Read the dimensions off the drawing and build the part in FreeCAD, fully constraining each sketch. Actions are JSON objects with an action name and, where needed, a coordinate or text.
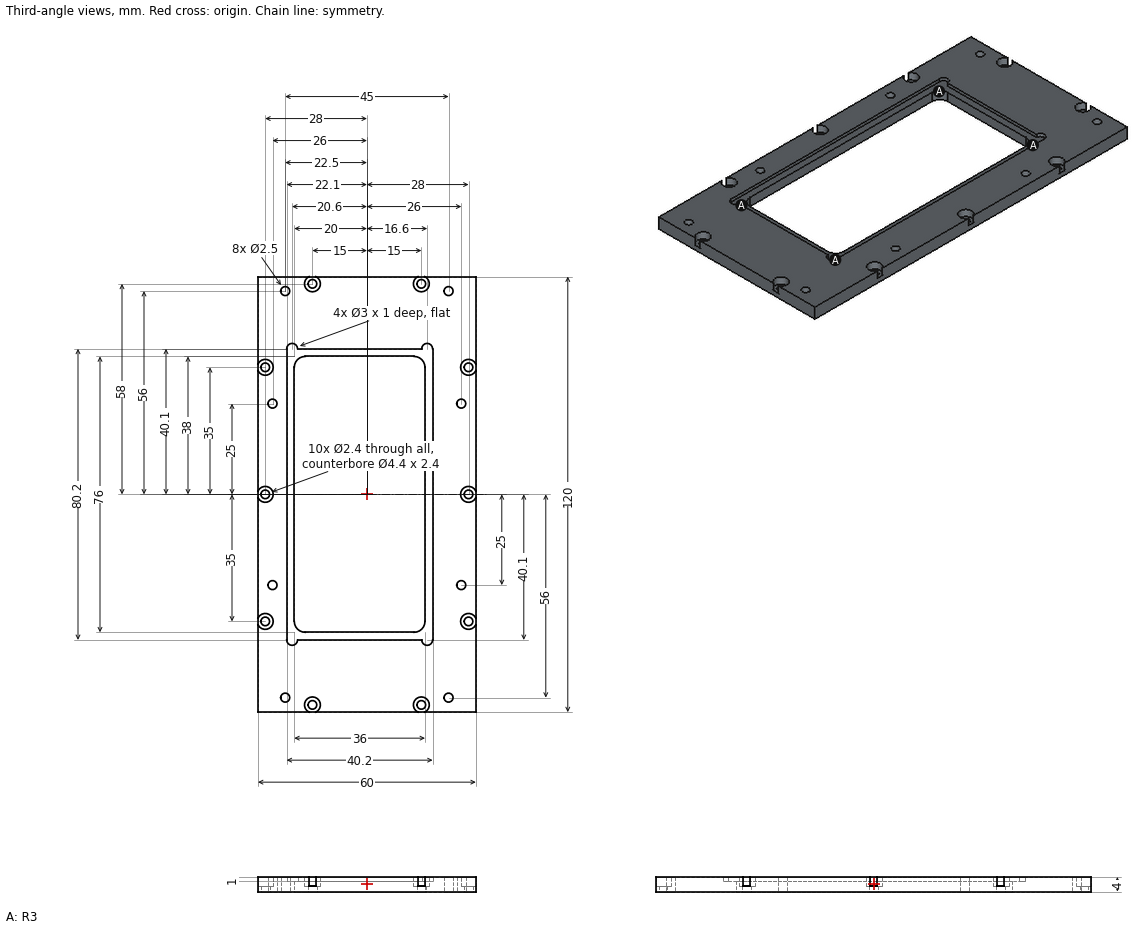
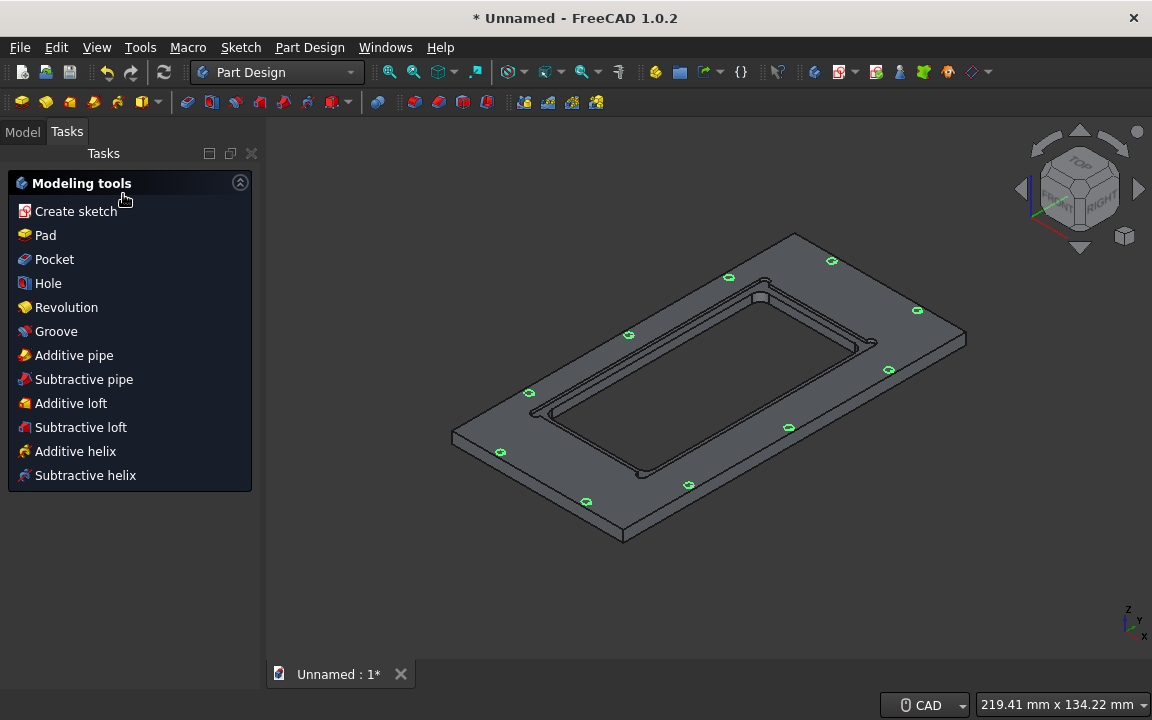
{"action": "left_click", "coordinate": [212, 102]}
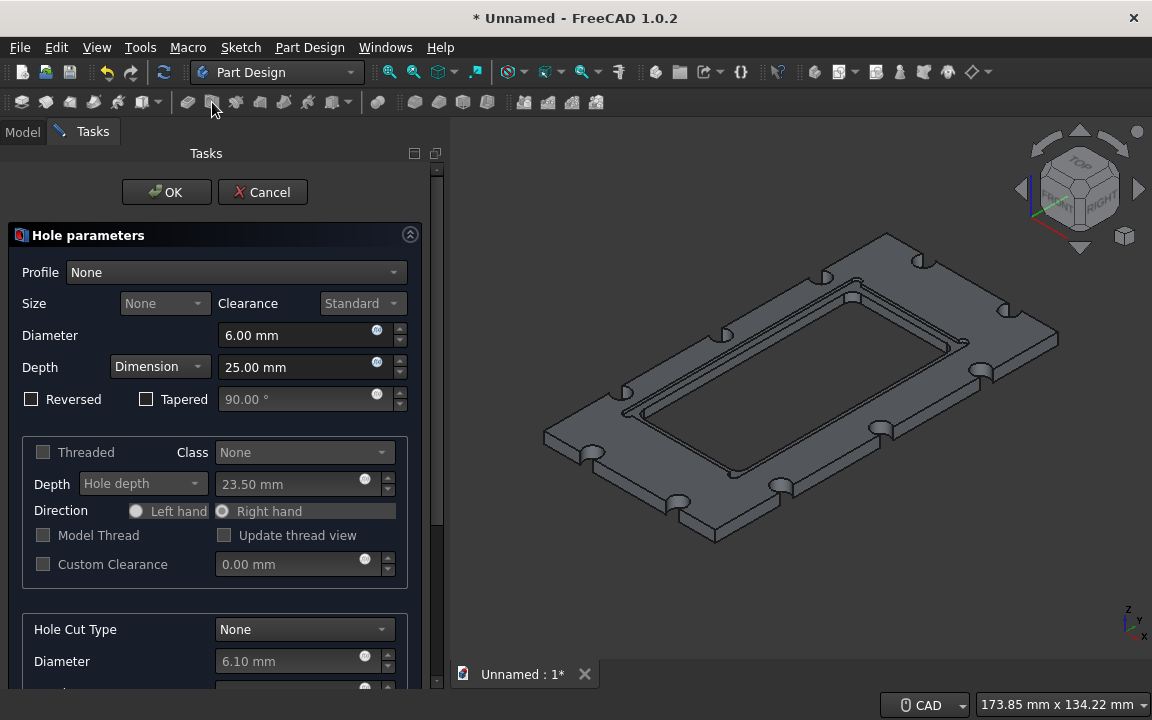
{"action": "triple_click", "coordinate": [305, 335]}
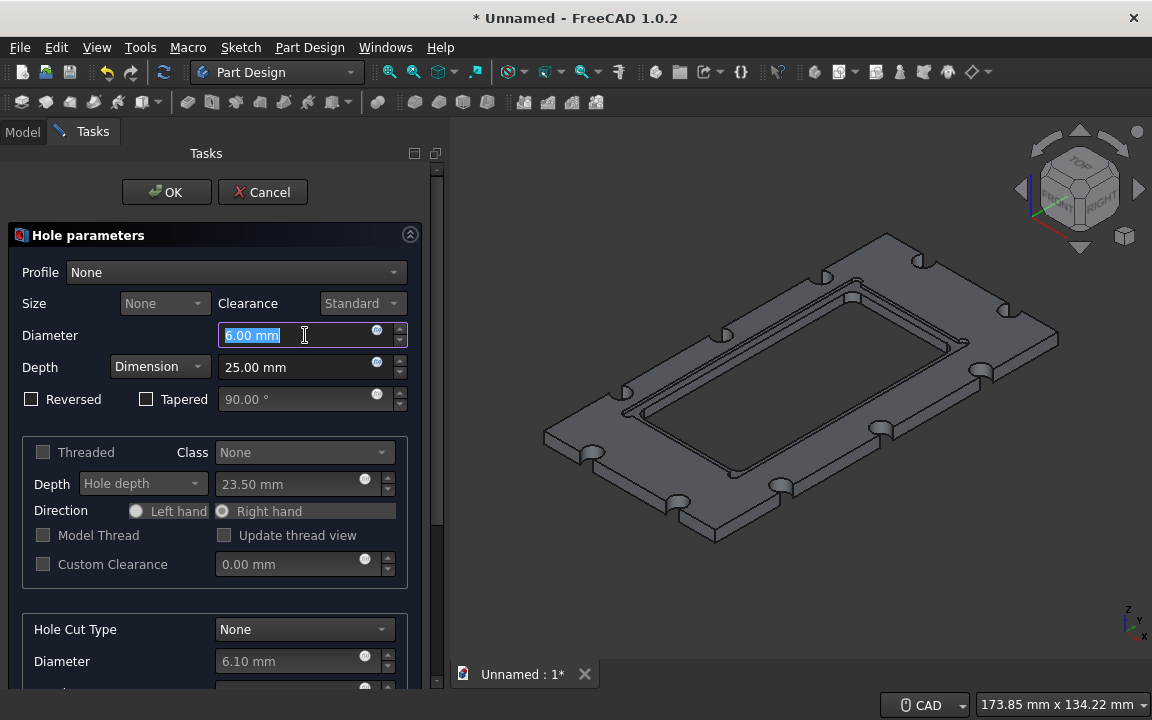
{"action": "type", "text": "2.4"}
{"action": "key", "text": "Tab"}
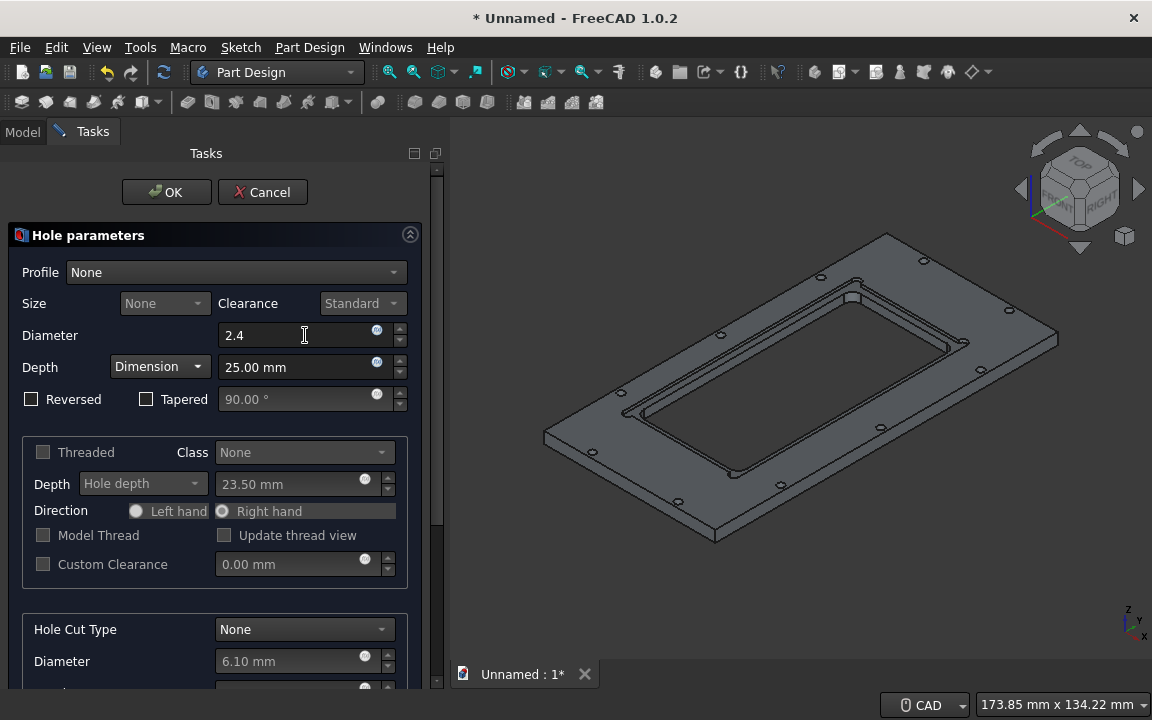
{"action": "left_click", "coordinate": [161, 366]}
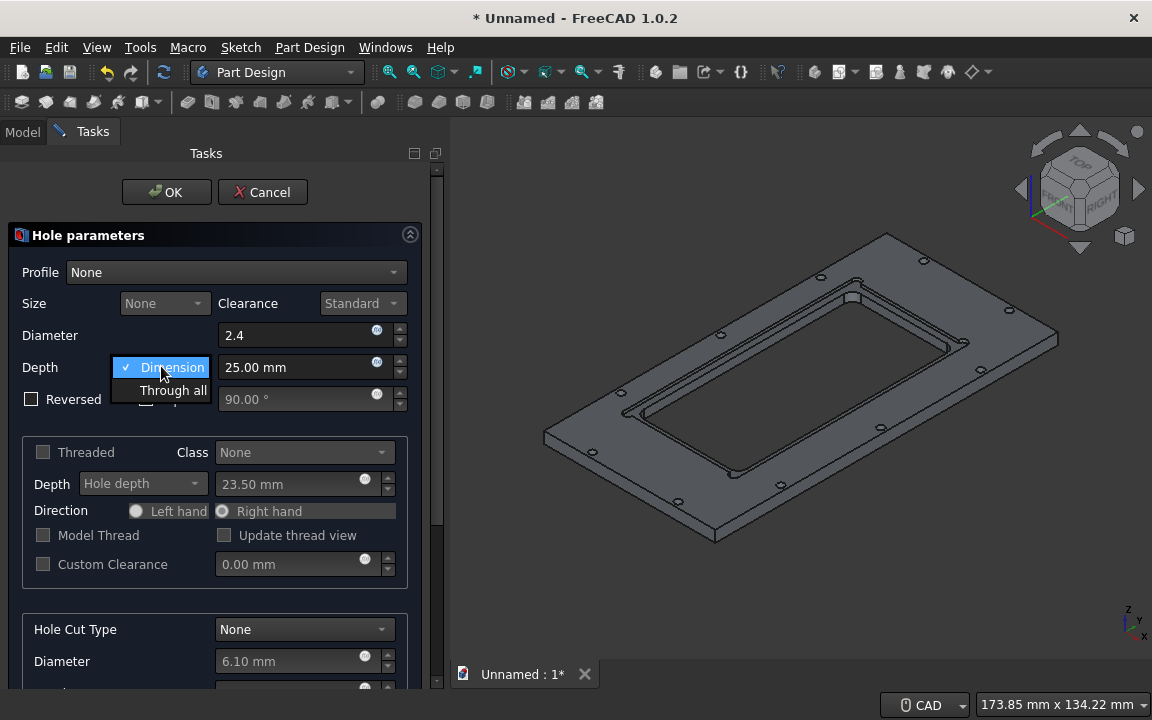
{"action": "left_click", "coordinate": [160, 390]}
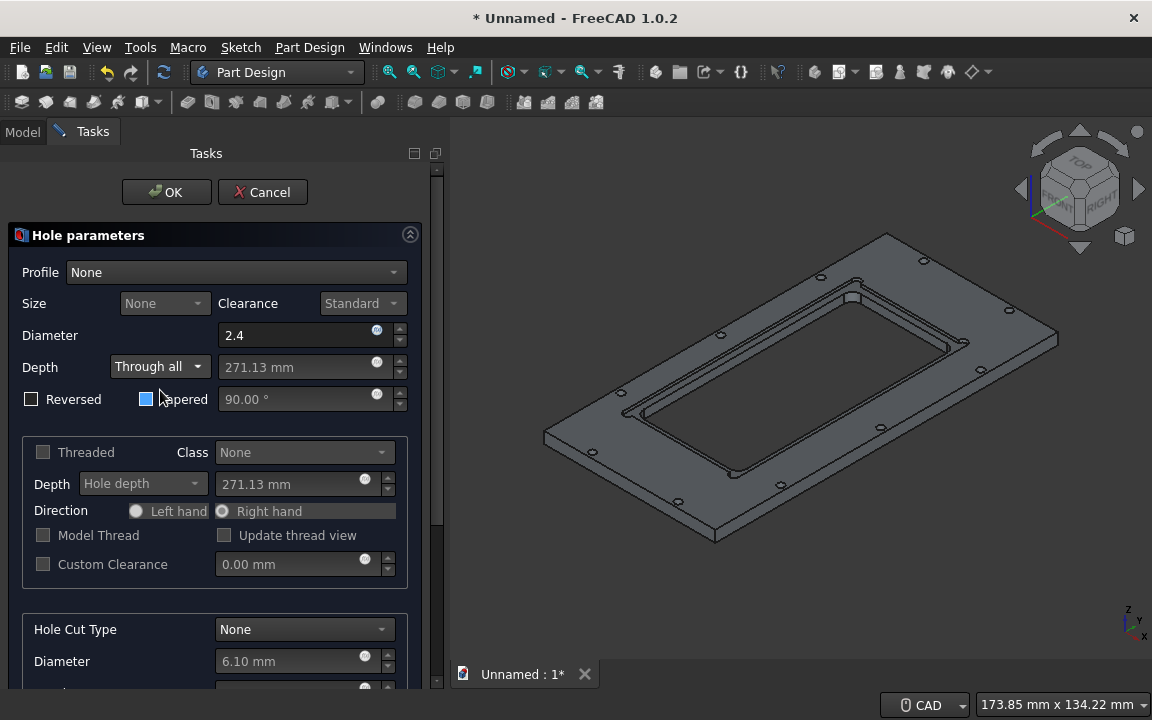
{"action": "left_click", "coordinate": [306, 630]}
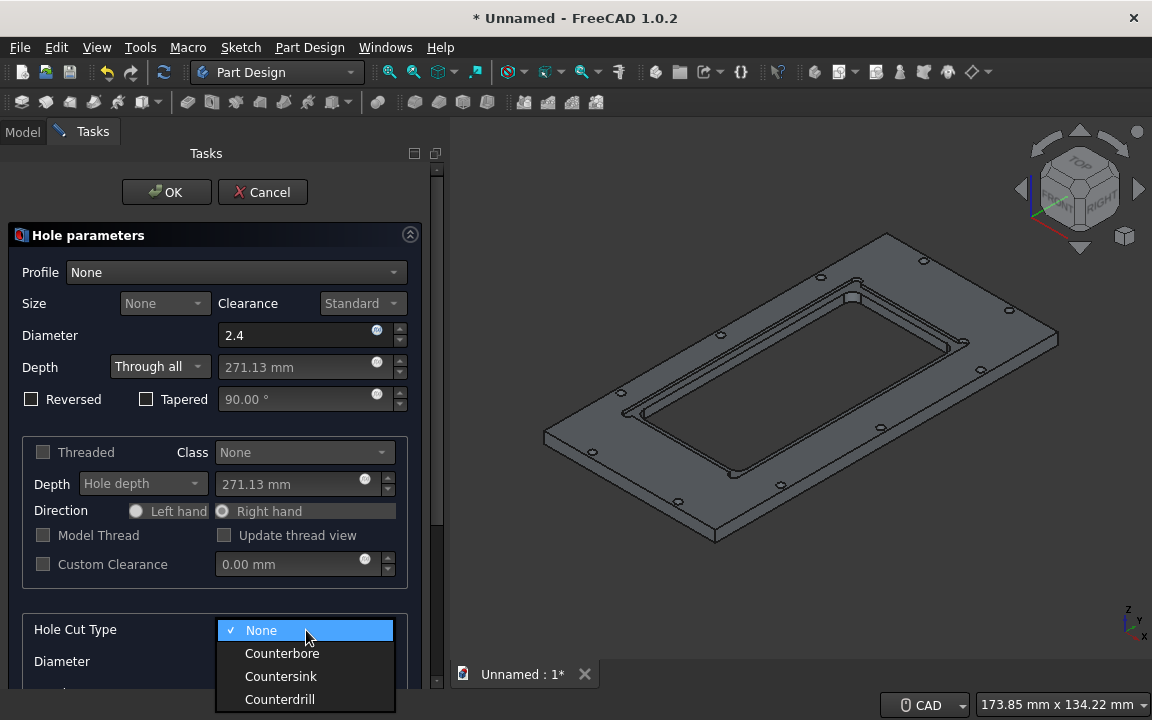
{"action": "left_click", "coordinate": [304, 654]}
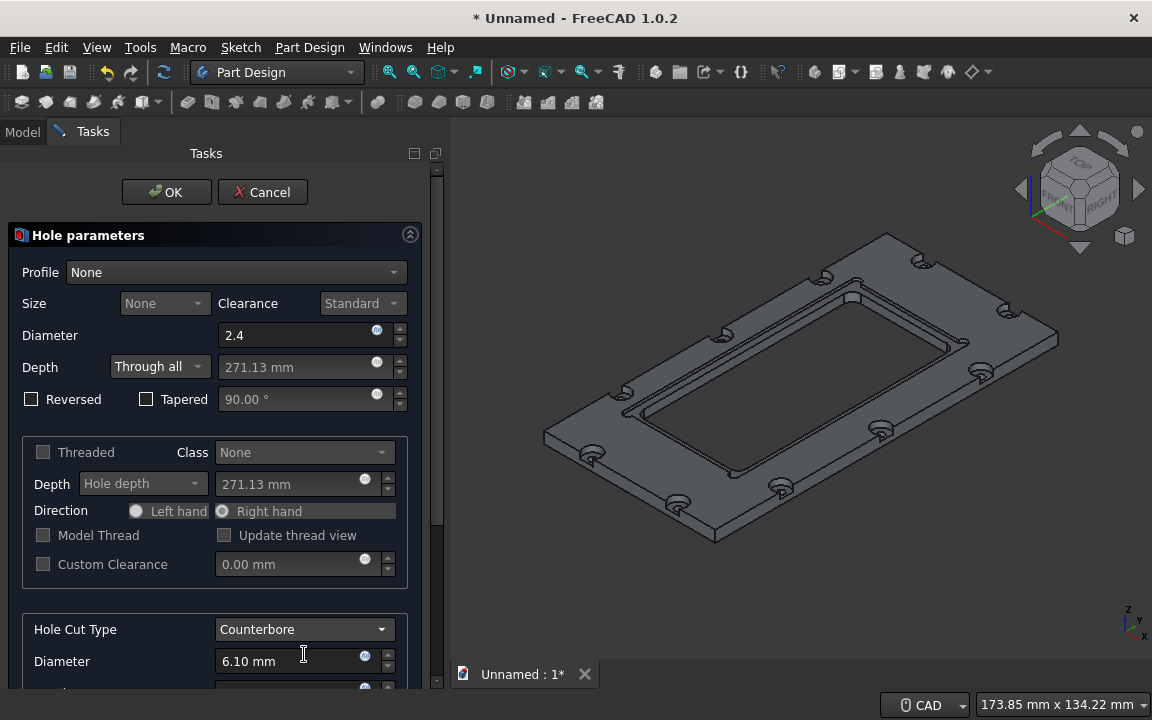
{"action": "triple_click", "coordinate": [298, 661]}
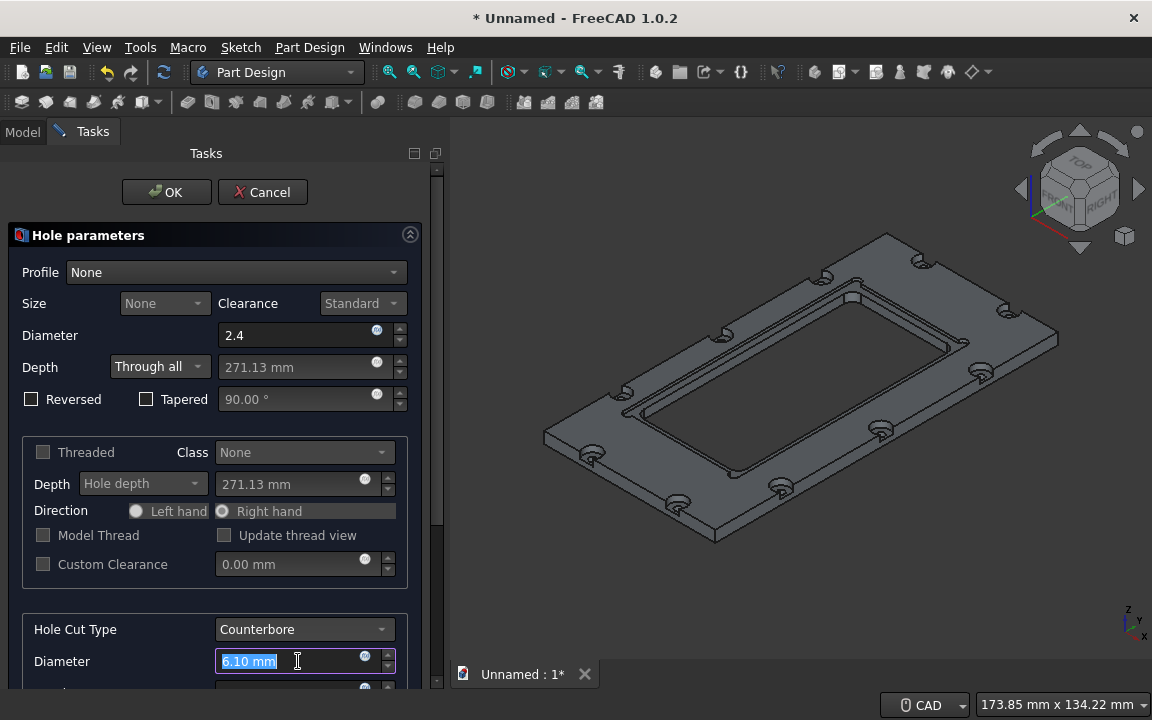
{"action": "type", "text": "4.4"}
{"action": "key", "text": "Tab"}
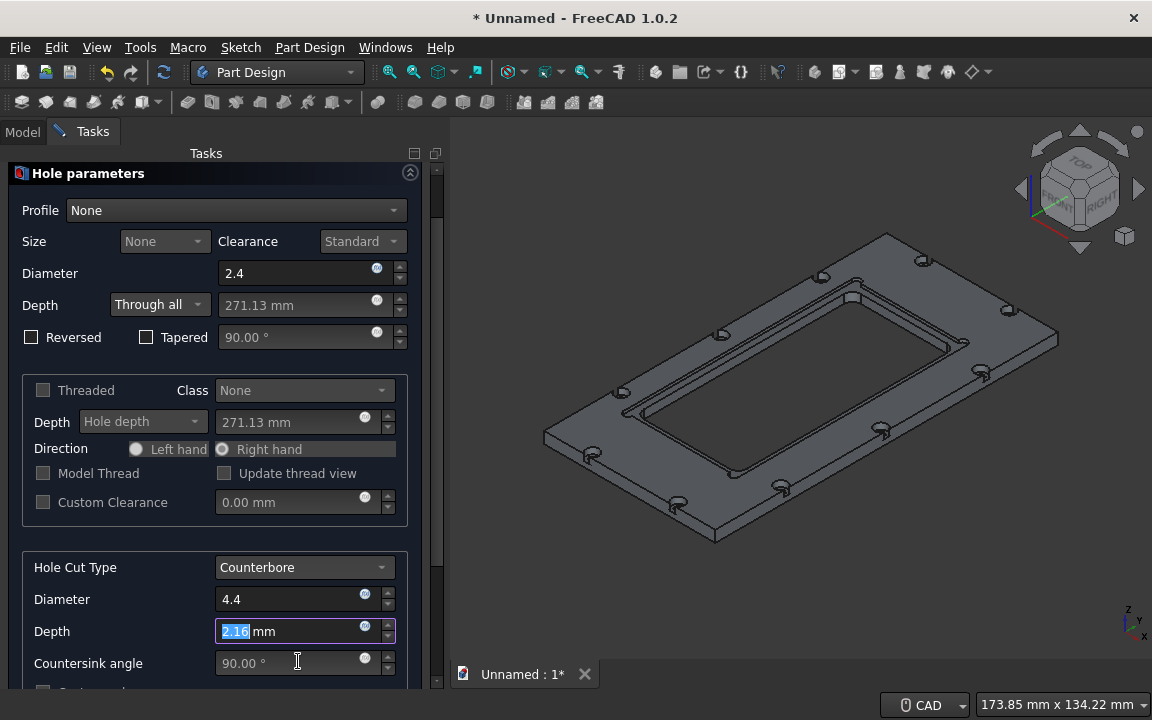
{"action": "type", "text": "2.4"}
{"action": "key", "text": "Tab"}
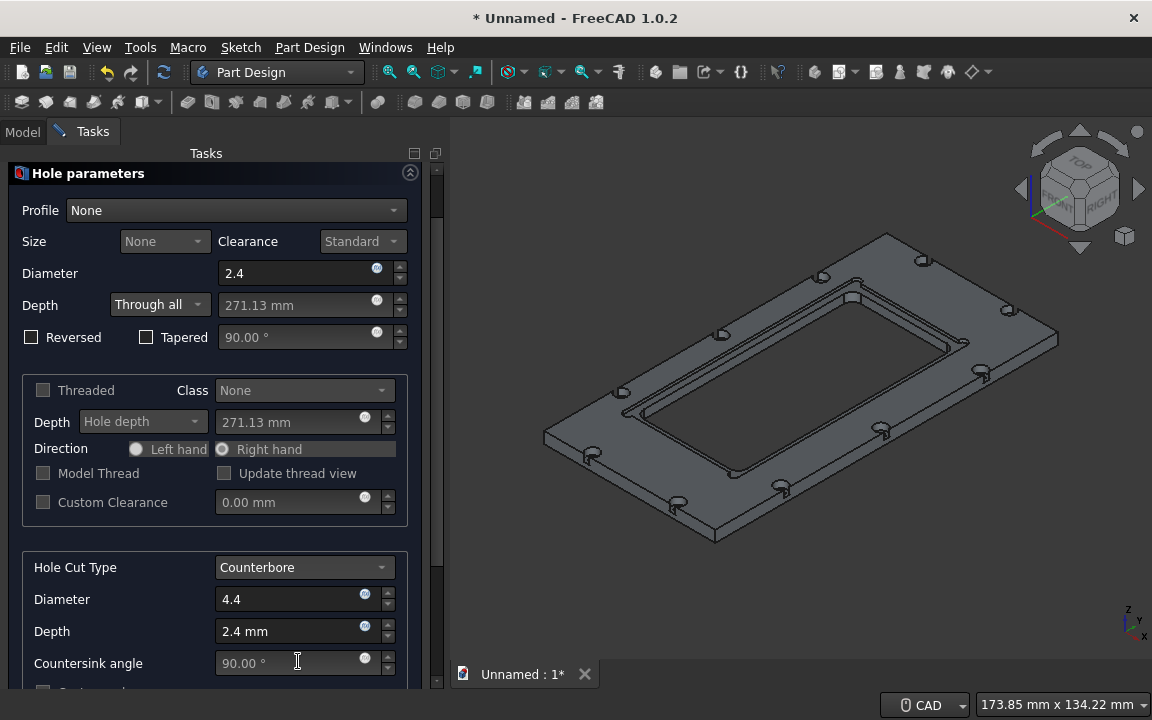
{"action": "scroll", "coordinate": [437, 426], "scroll_direction": "up", "scroll_amount": 2}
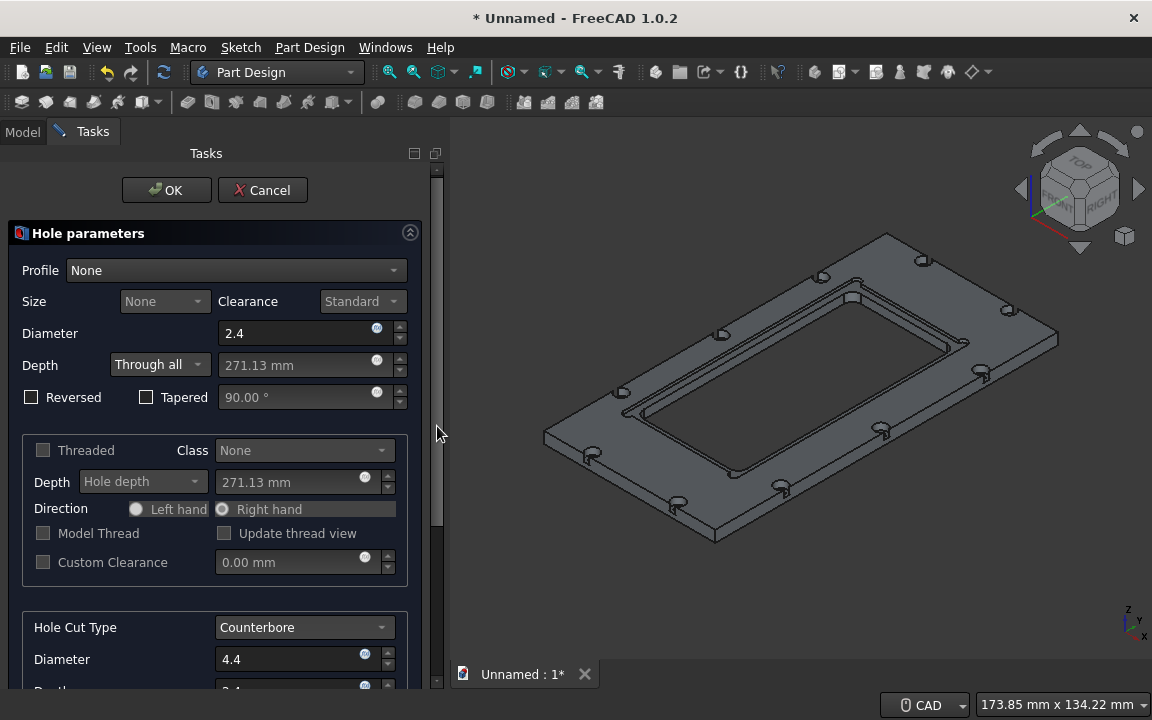
{"action": "left_click", "coordinate": [167, 192]}